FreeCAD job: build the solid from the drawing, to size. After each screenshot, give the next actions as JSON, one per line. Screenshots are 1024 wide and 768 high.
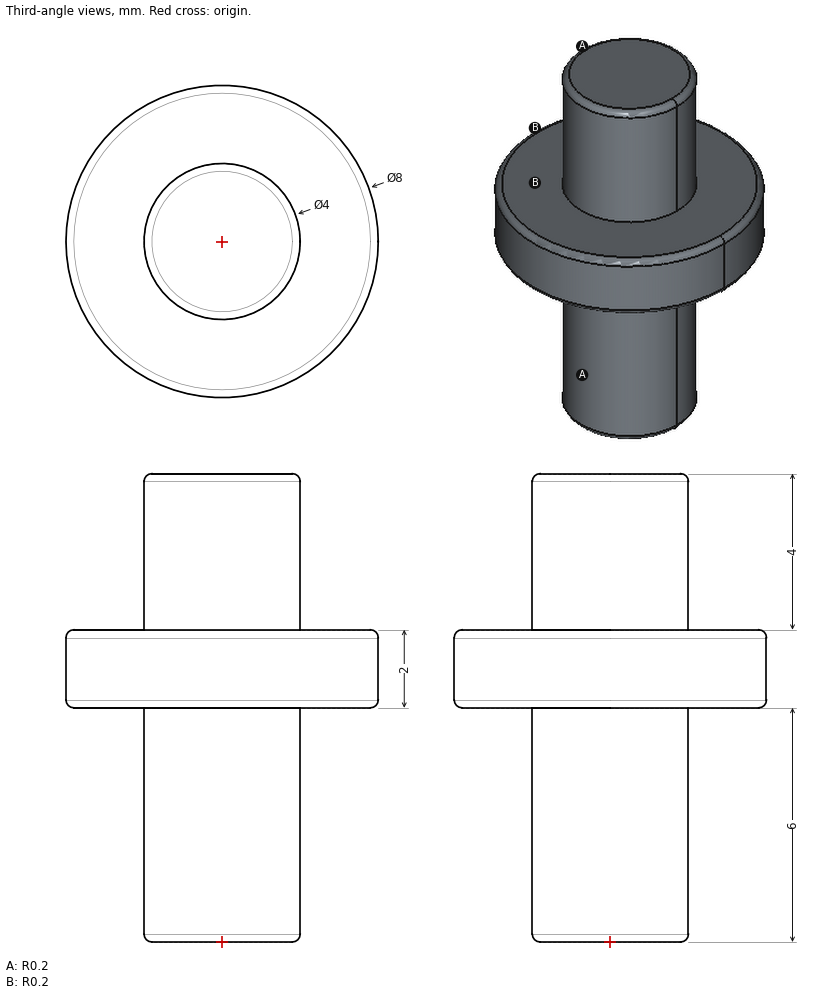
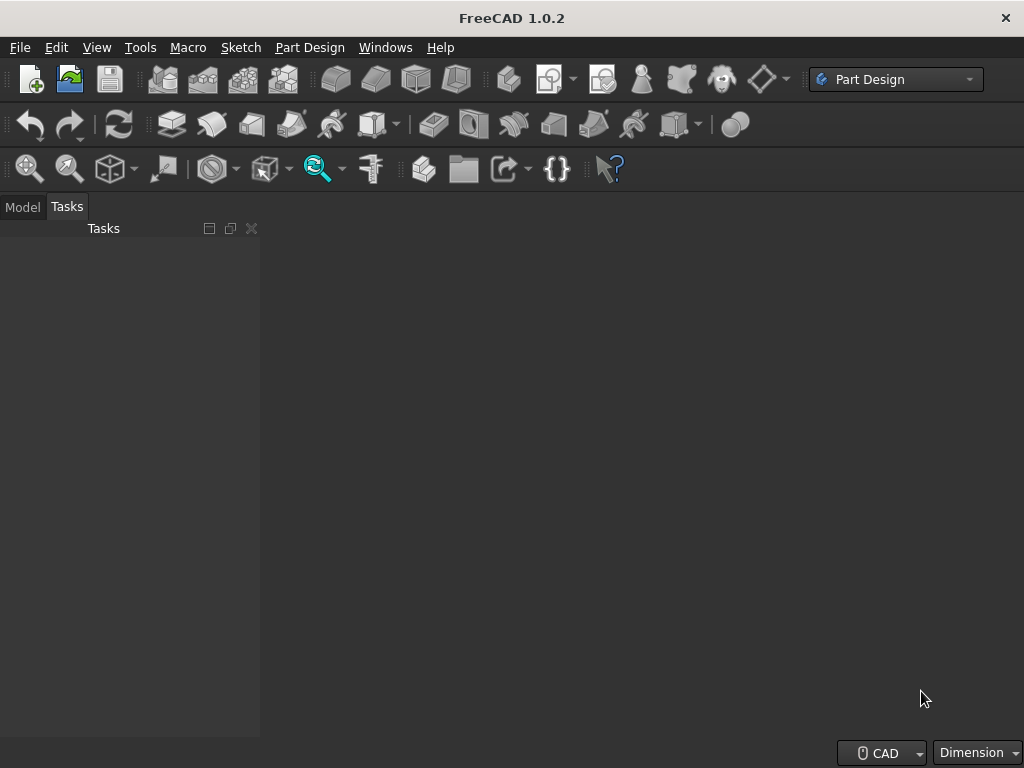
{"action": "left_click", "coordinate": [30, 80]}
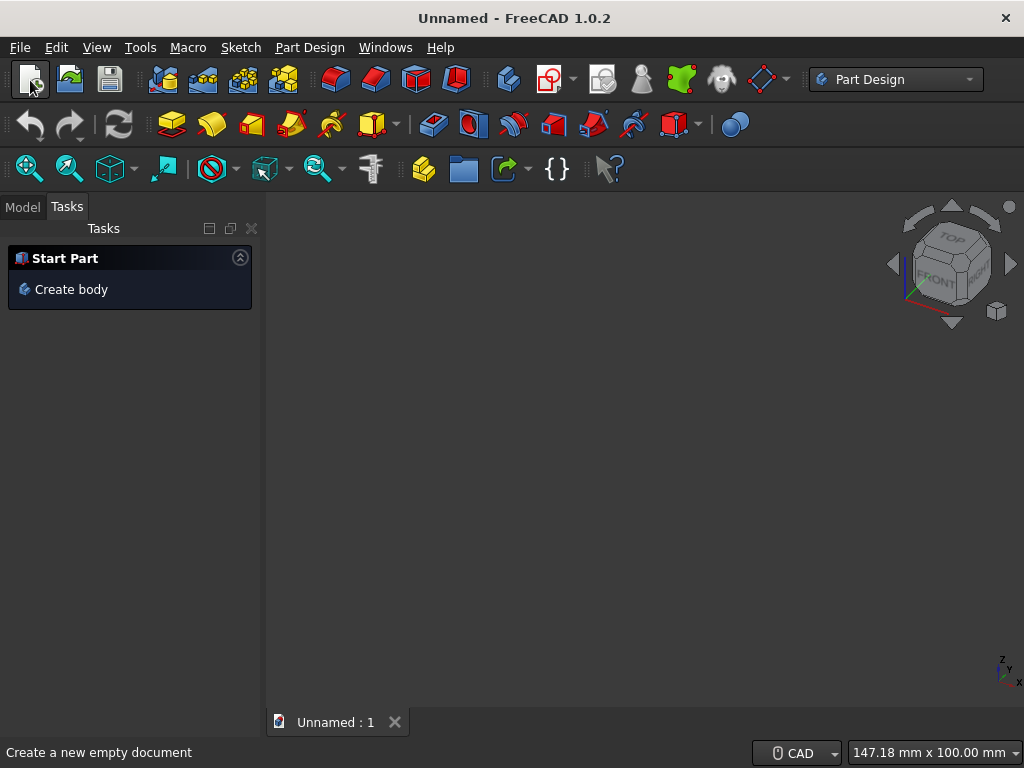
{"action": "left_click", "coordinate": [550, 80]}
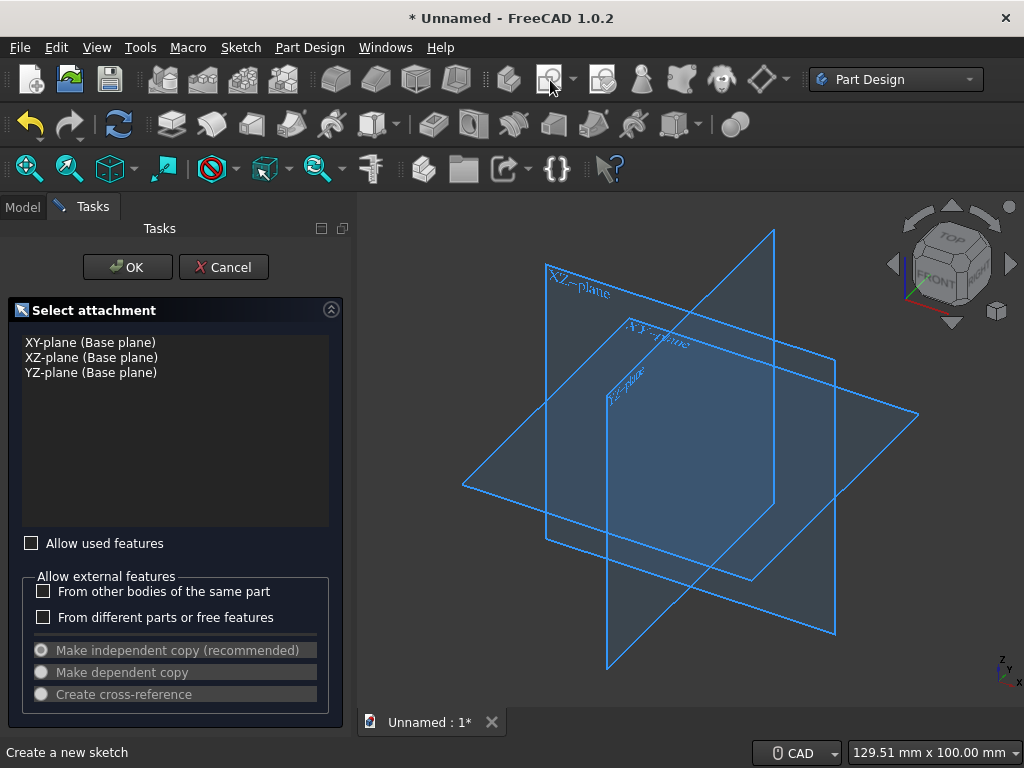
{"action": "left_click", "coordinate": [82, 342]}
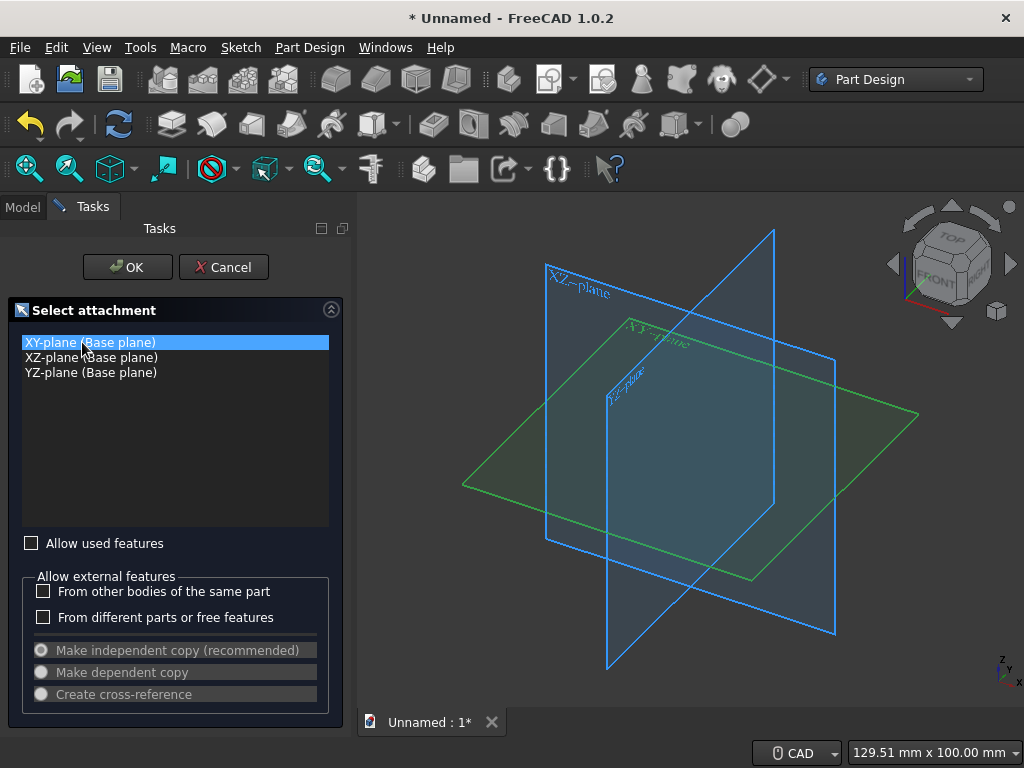
{"action": "left_click", "coordinate": [128, 267]}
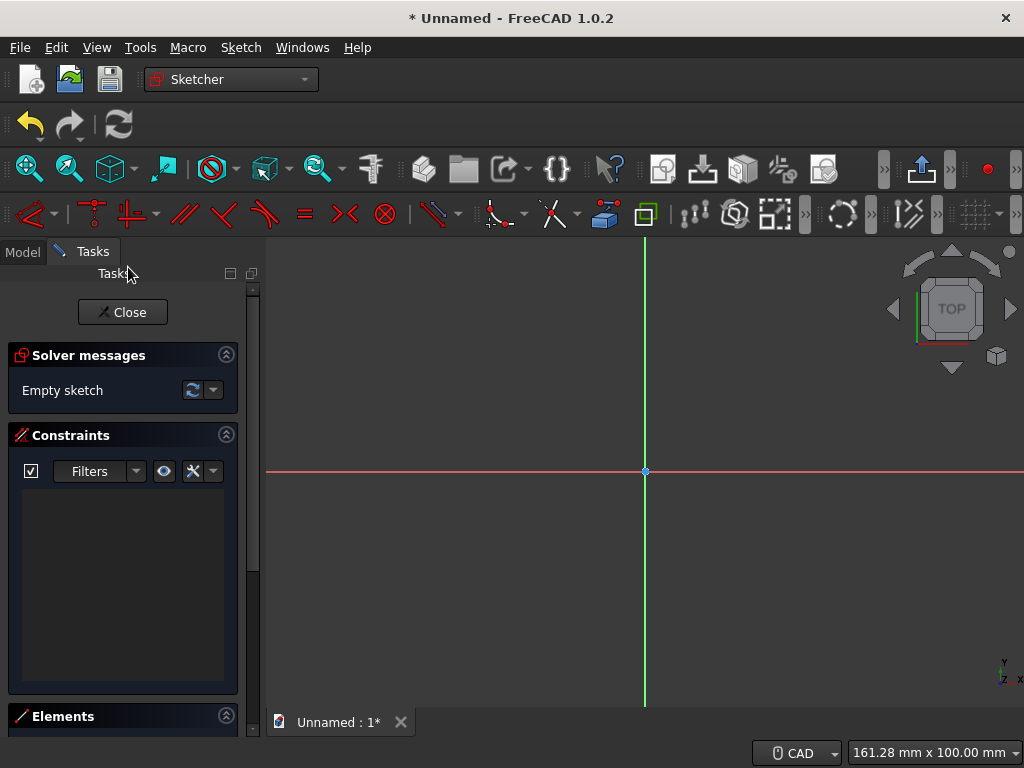
{"action": "scroll", "coordinate": [649, 472], "scroll_direction": "up", "scroll_amount": 14}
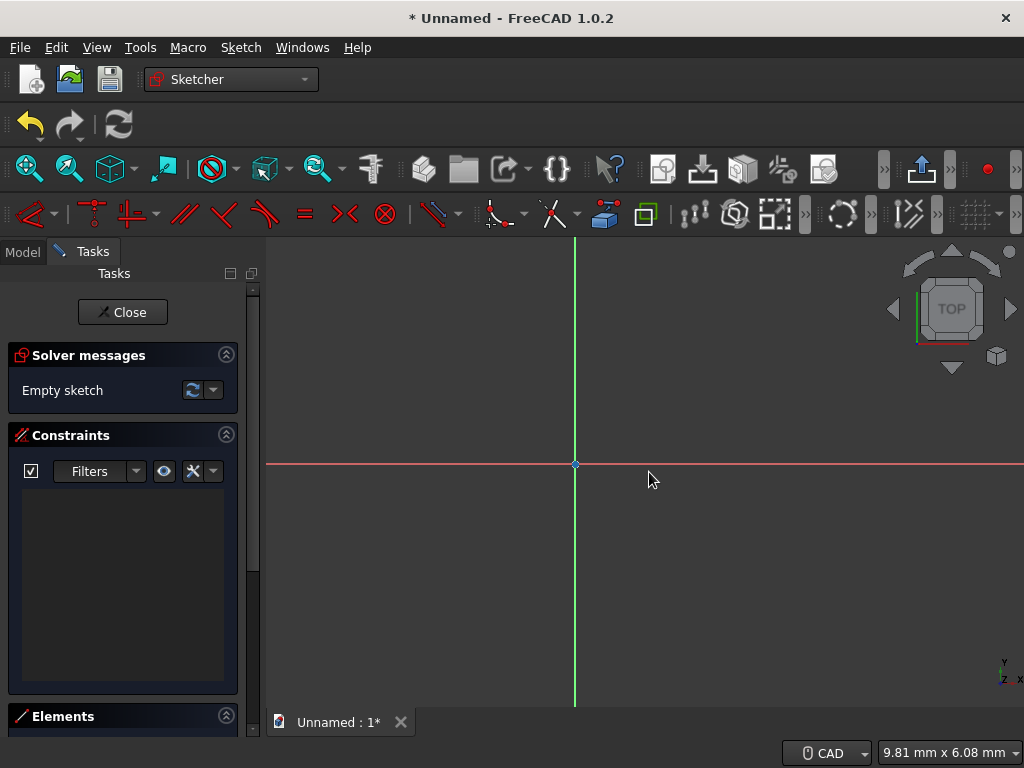
{"action": "key", "text": "g c"}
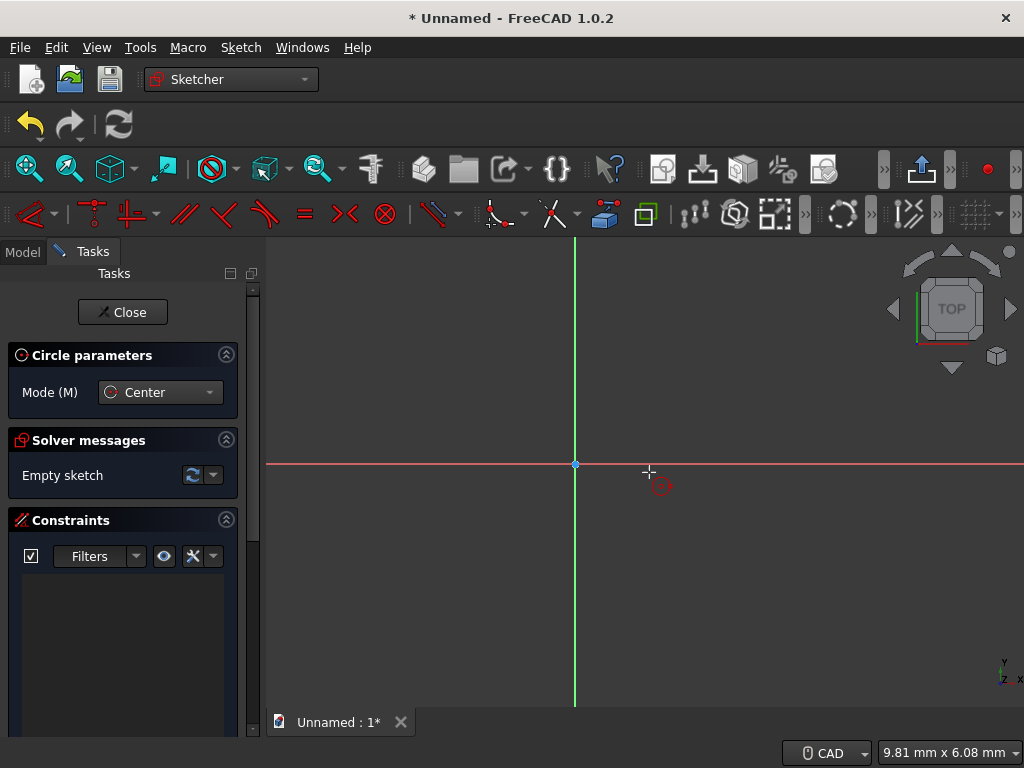
{"action": "left_click", "coordinate": [575, 464]}
{"action": "left_click", "coordinate": [685, 355]}
{"action": "key", "text": "Escape"}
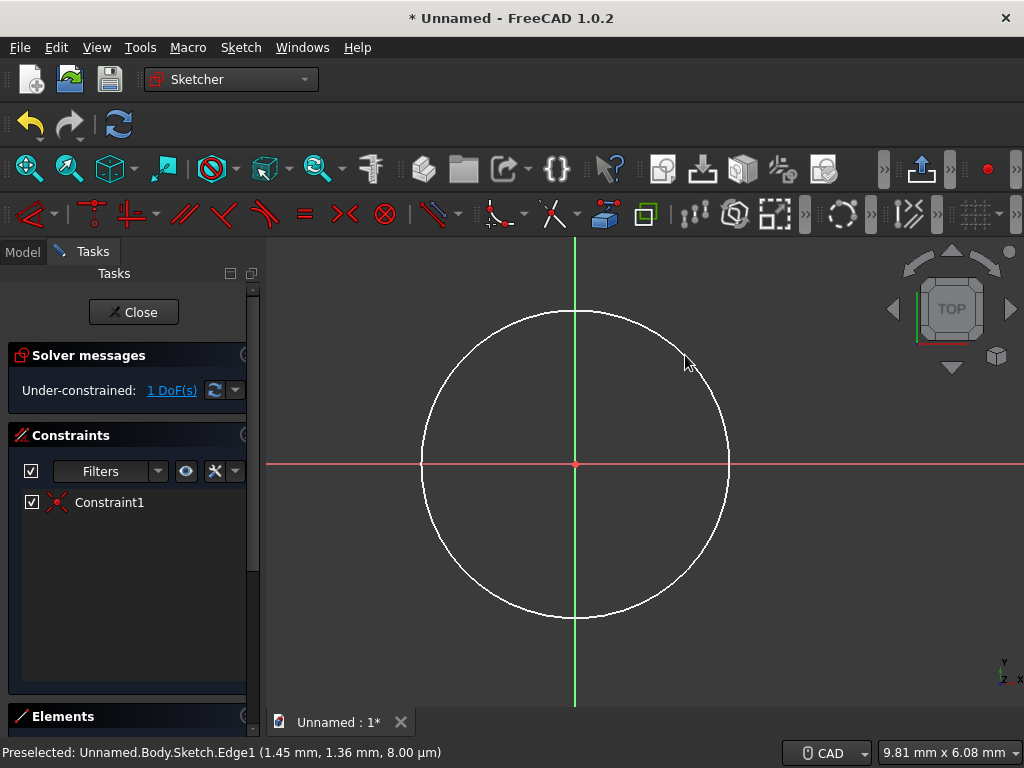
{"action": "left_click", "coordinate": [30, 214]}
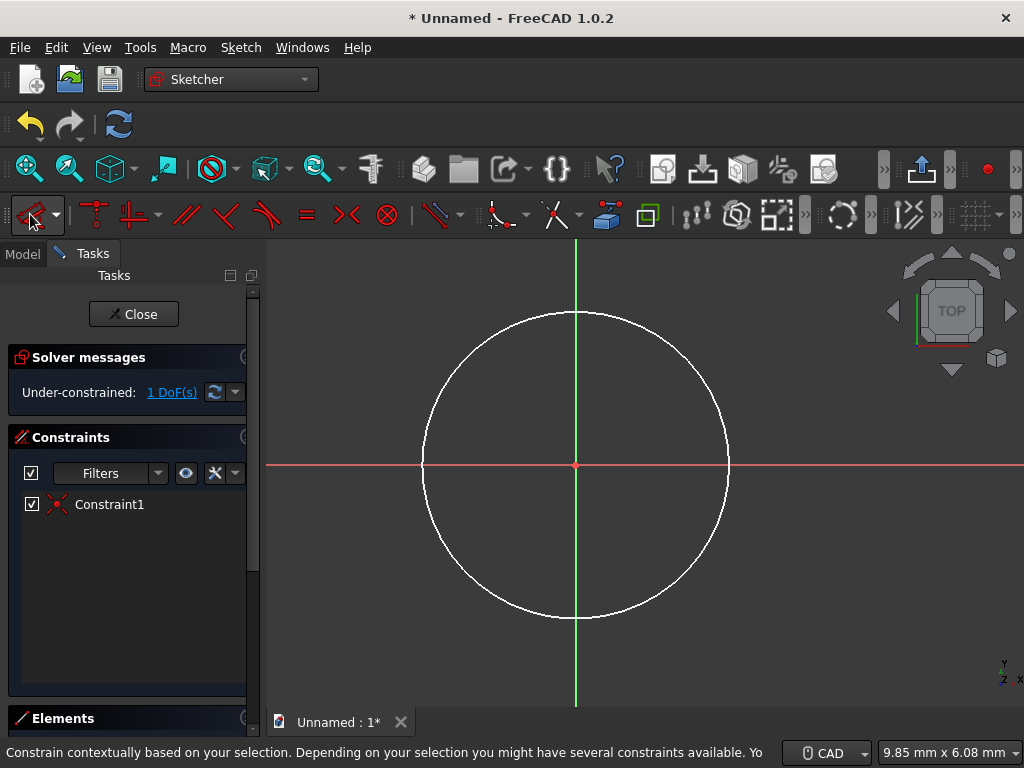
{"action": "left_click", "coordinate": [684, 356]}
{"action": "left_click", "coordinate": [707, 333]}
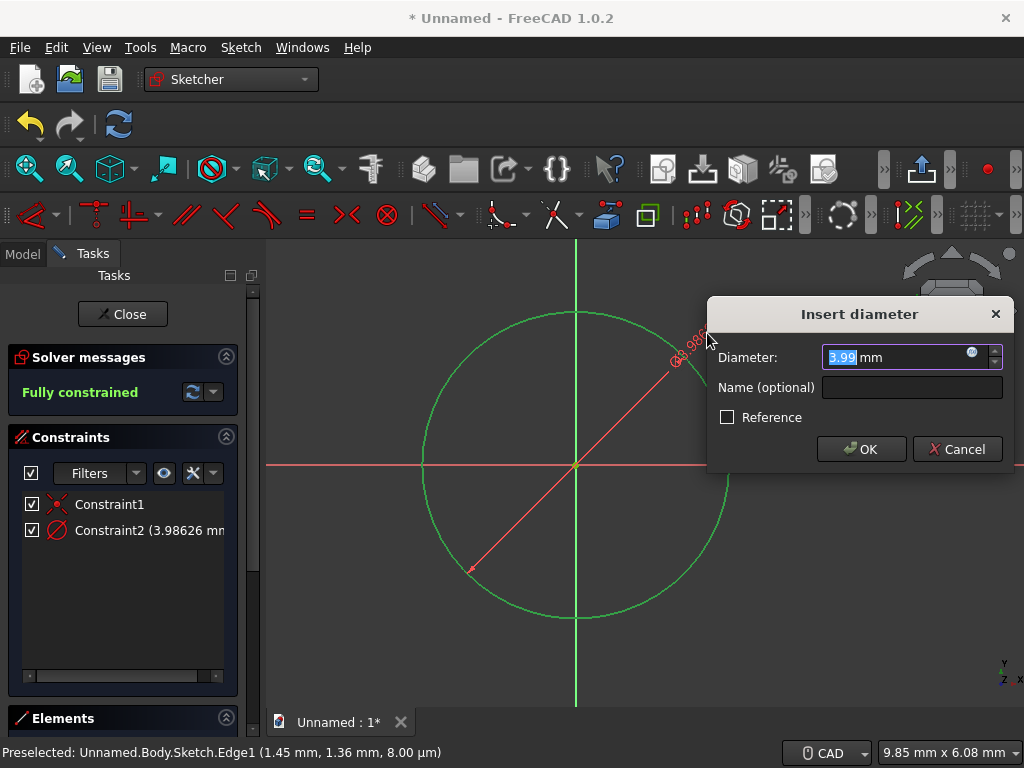
{"action": "type", "text": "4"}
{"action": "key", "text": "Return"}
{"action": "key", "text": "Escape"}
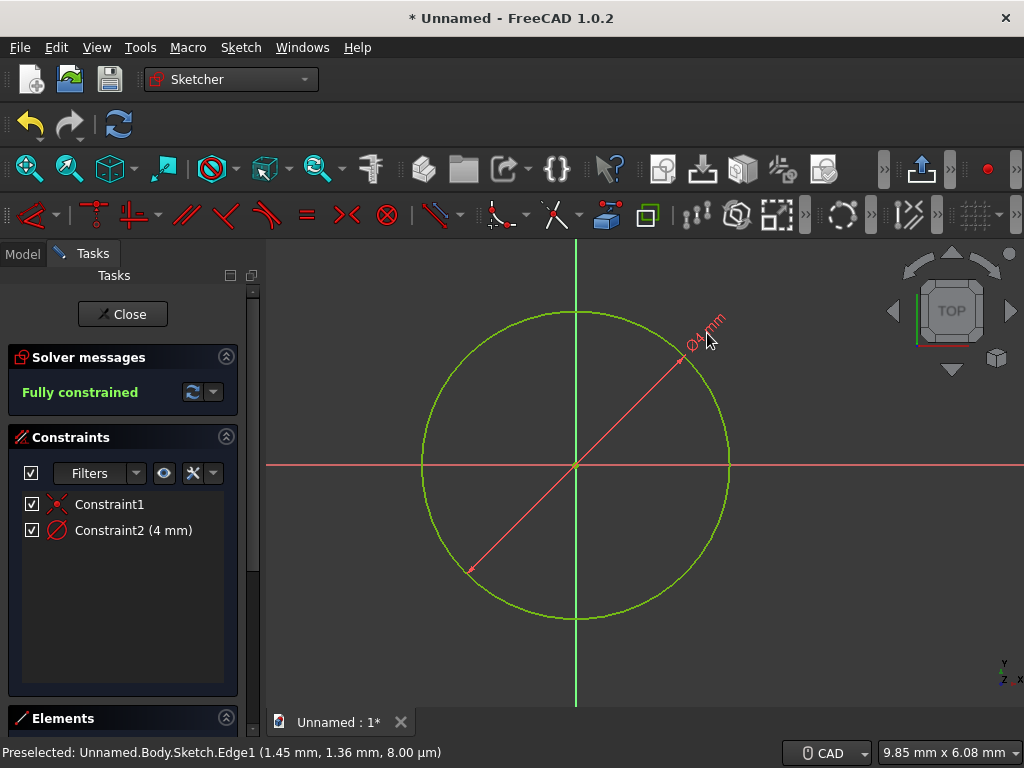
{"action": "left_click", "coordinate": [123, 314]}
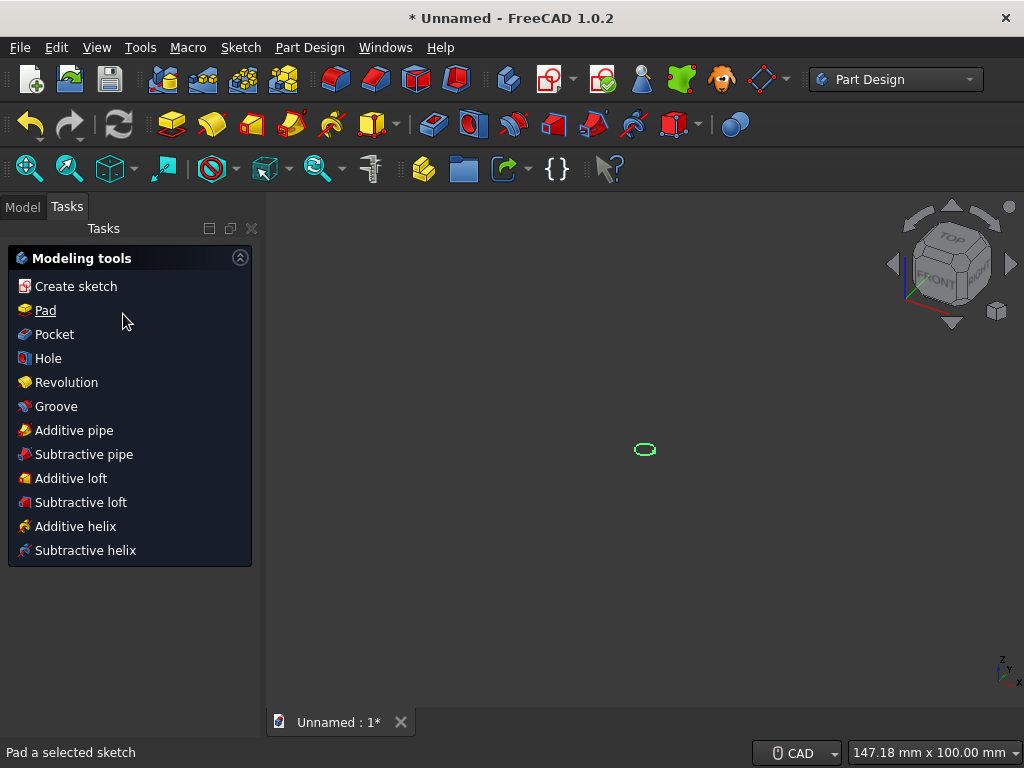
{"action": "left_click", "coordinate": [172, 124]}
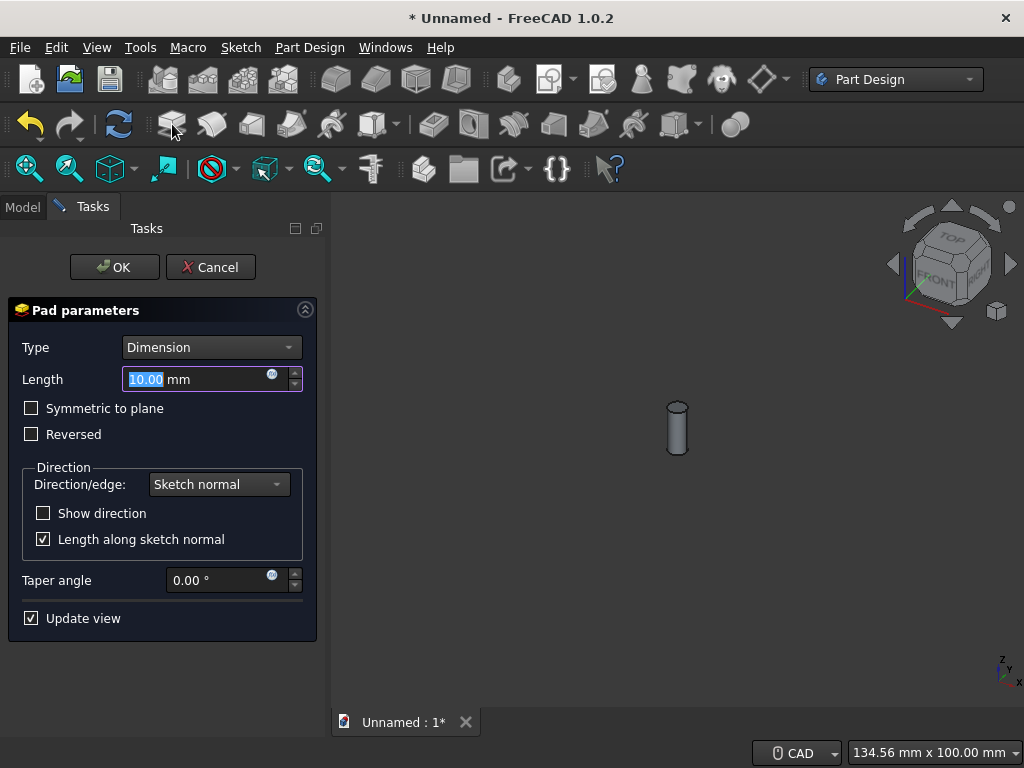
{"action": "type", "text": "6"}
{"action": "key", "text": "Tab"}